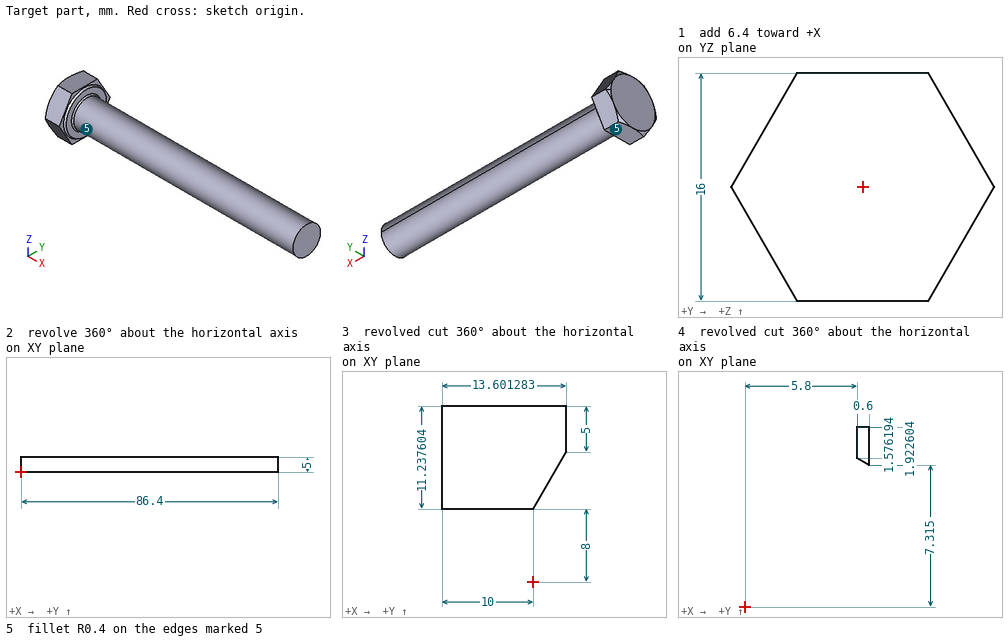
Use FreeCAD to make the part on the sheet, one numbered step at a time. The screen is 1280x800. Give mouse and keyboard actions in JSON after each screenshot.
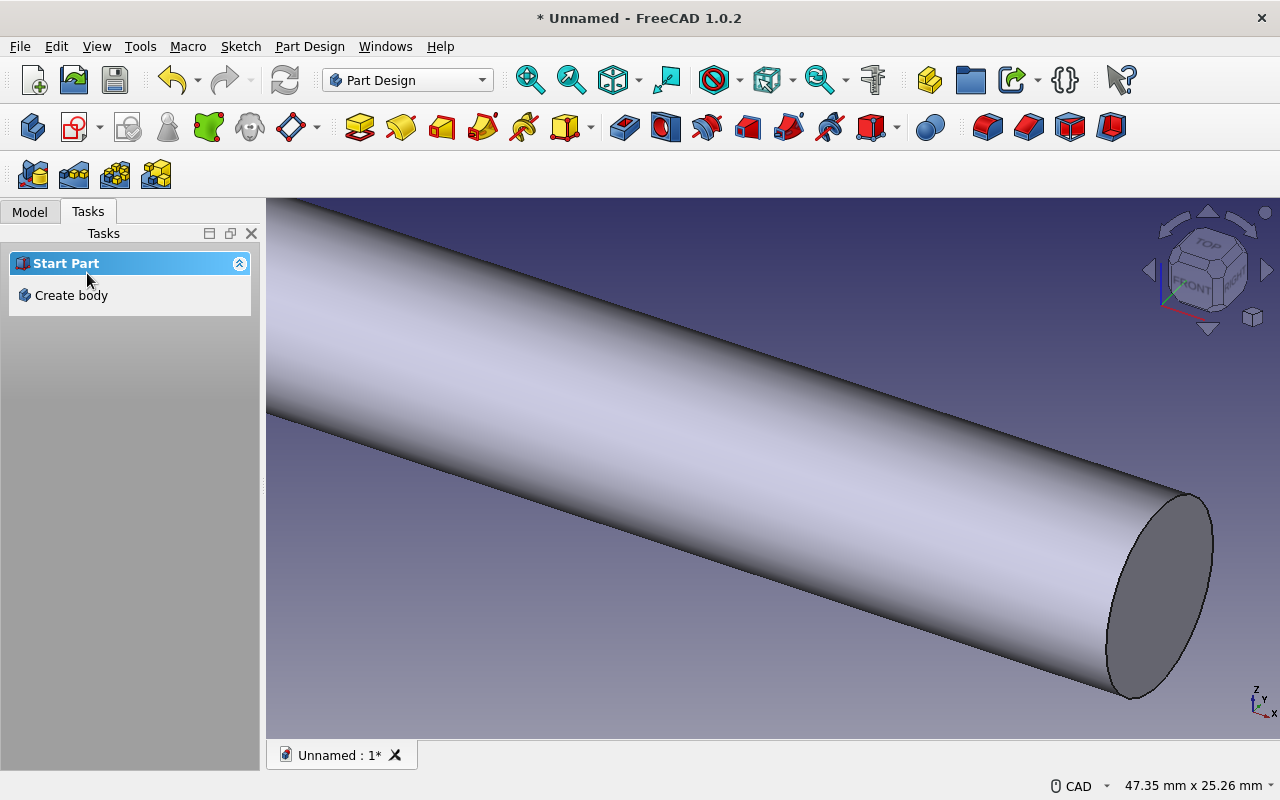
{"action": "key", "text": "v f"}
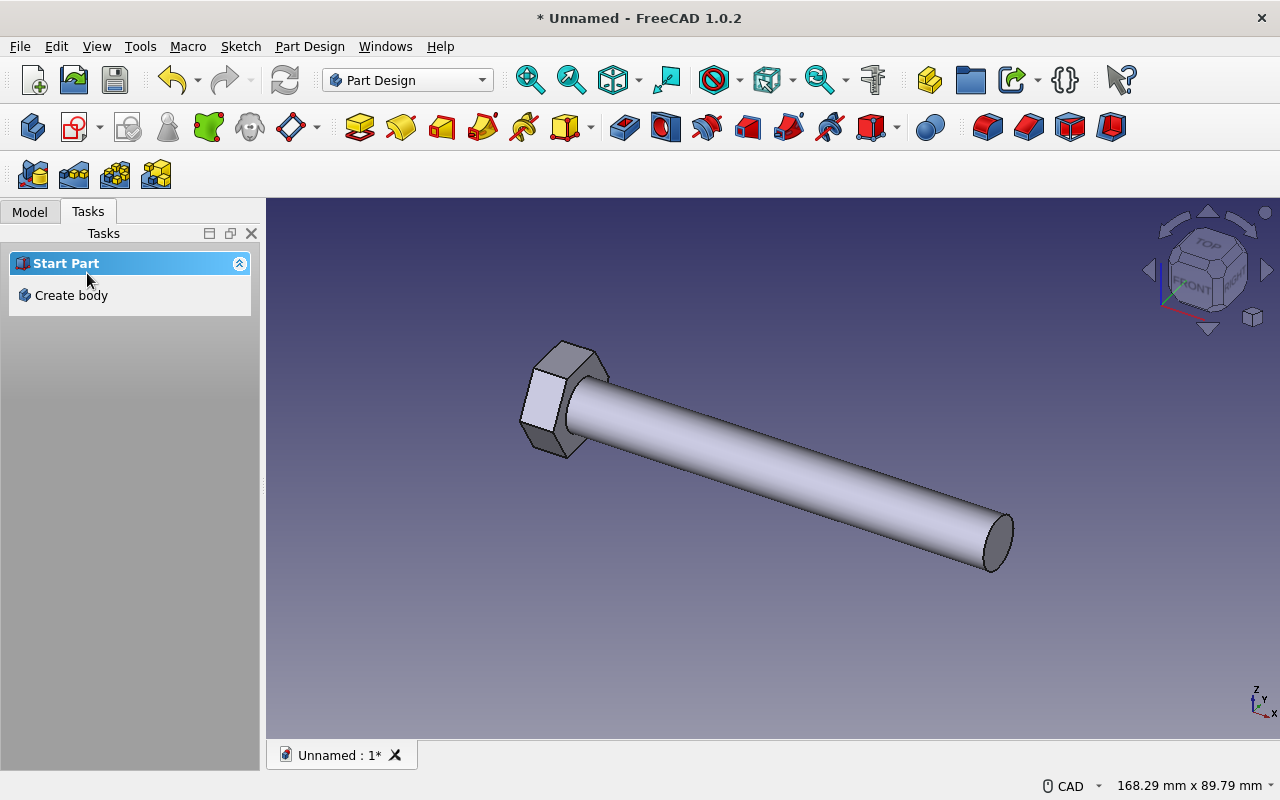
{"action": "left_click", "coordinate": [74, 128]}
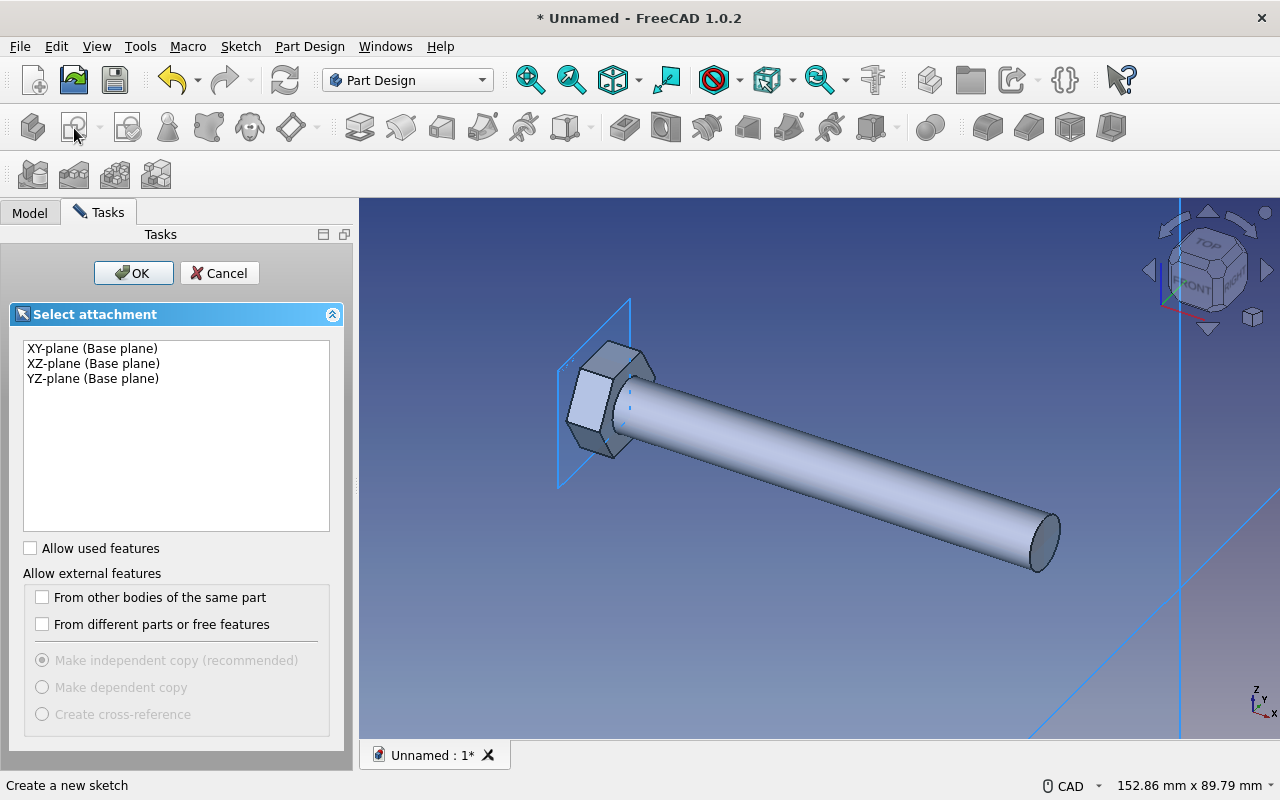
{"action": "left_click", "coordinate": [84, 348]}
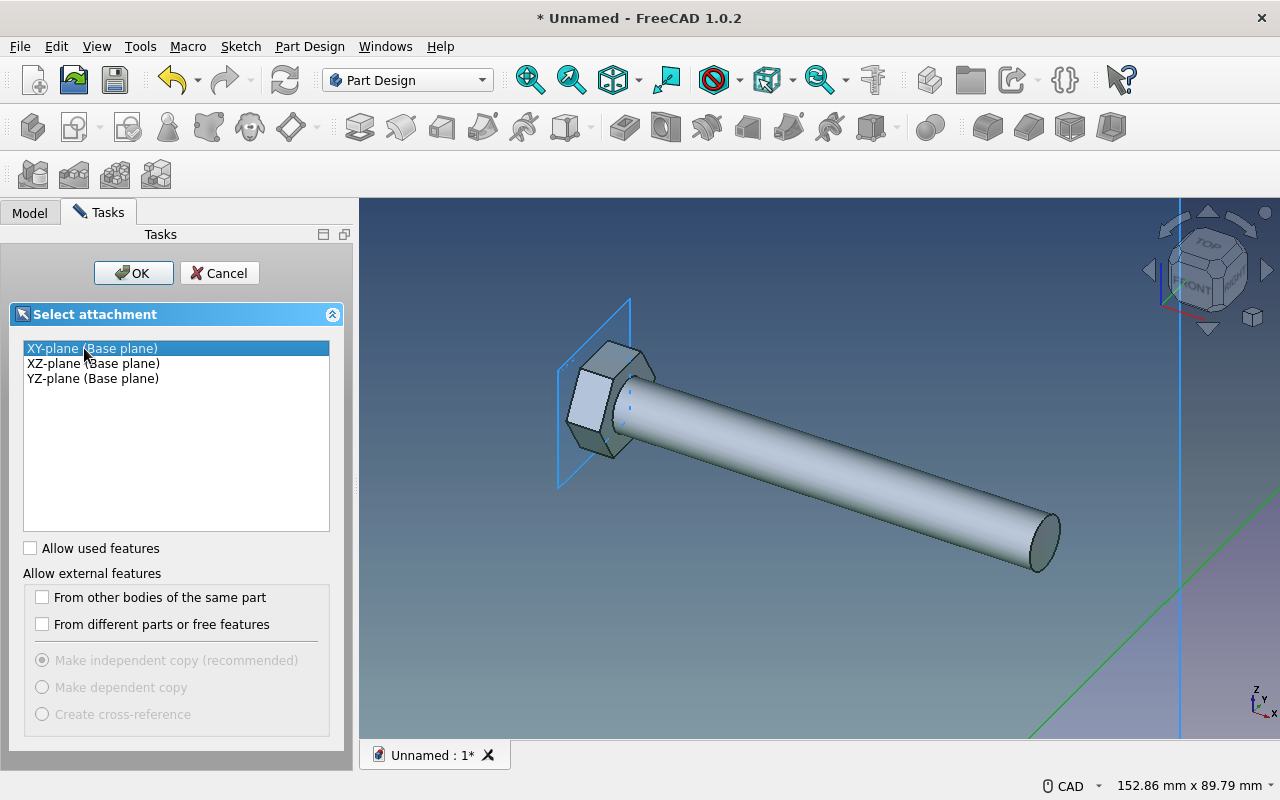
{"action": "left_click", "coordinate": [134, 273]}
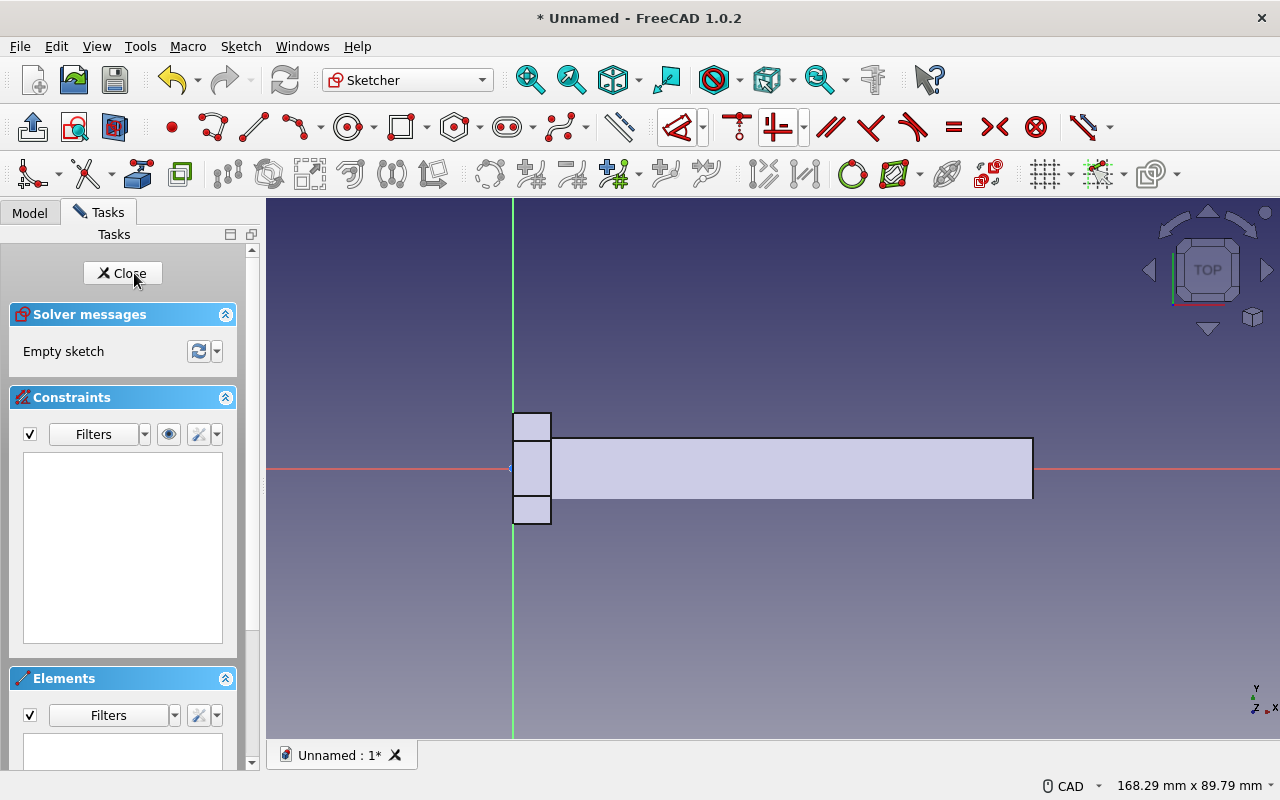
{"action": "left_click", "coordinate": [115, 128]}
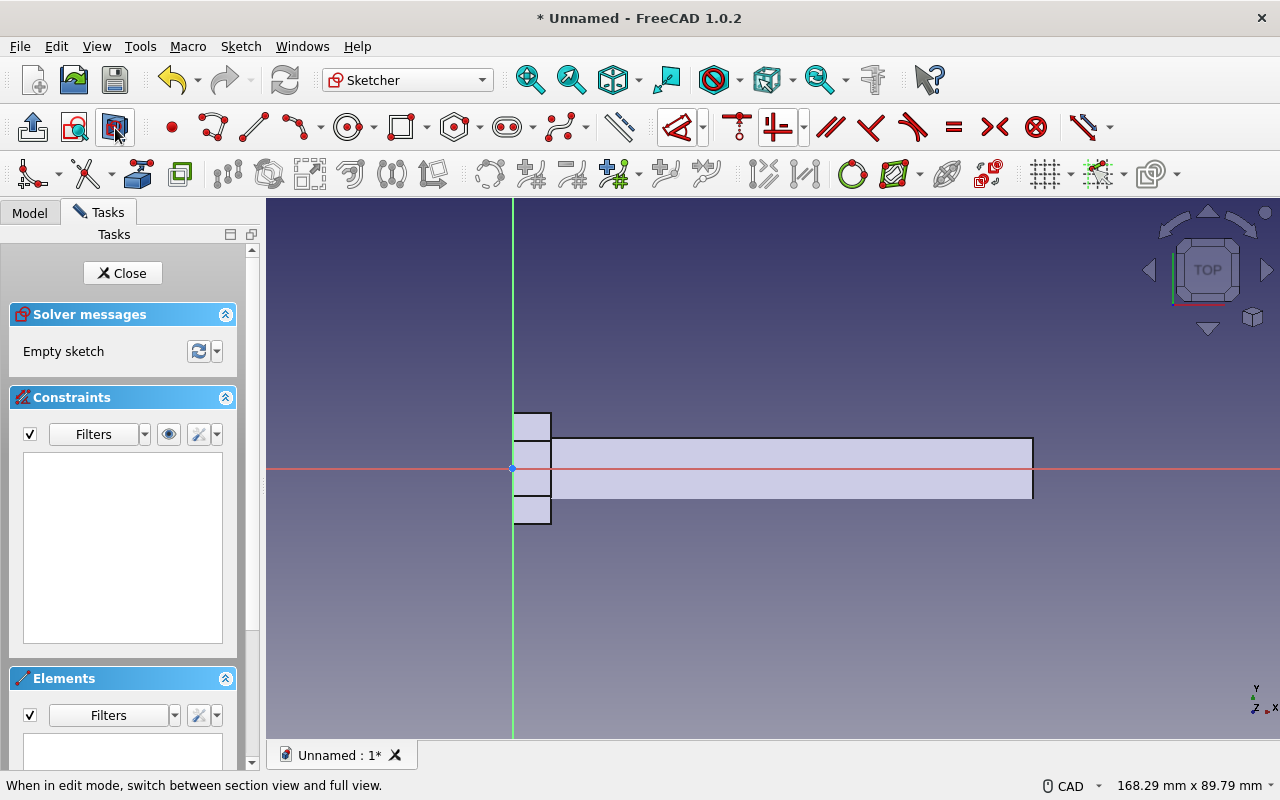
{"action": "scroll", "coordinate": [371, 377], "scroll_direction": "up", "scroll_amount": 5}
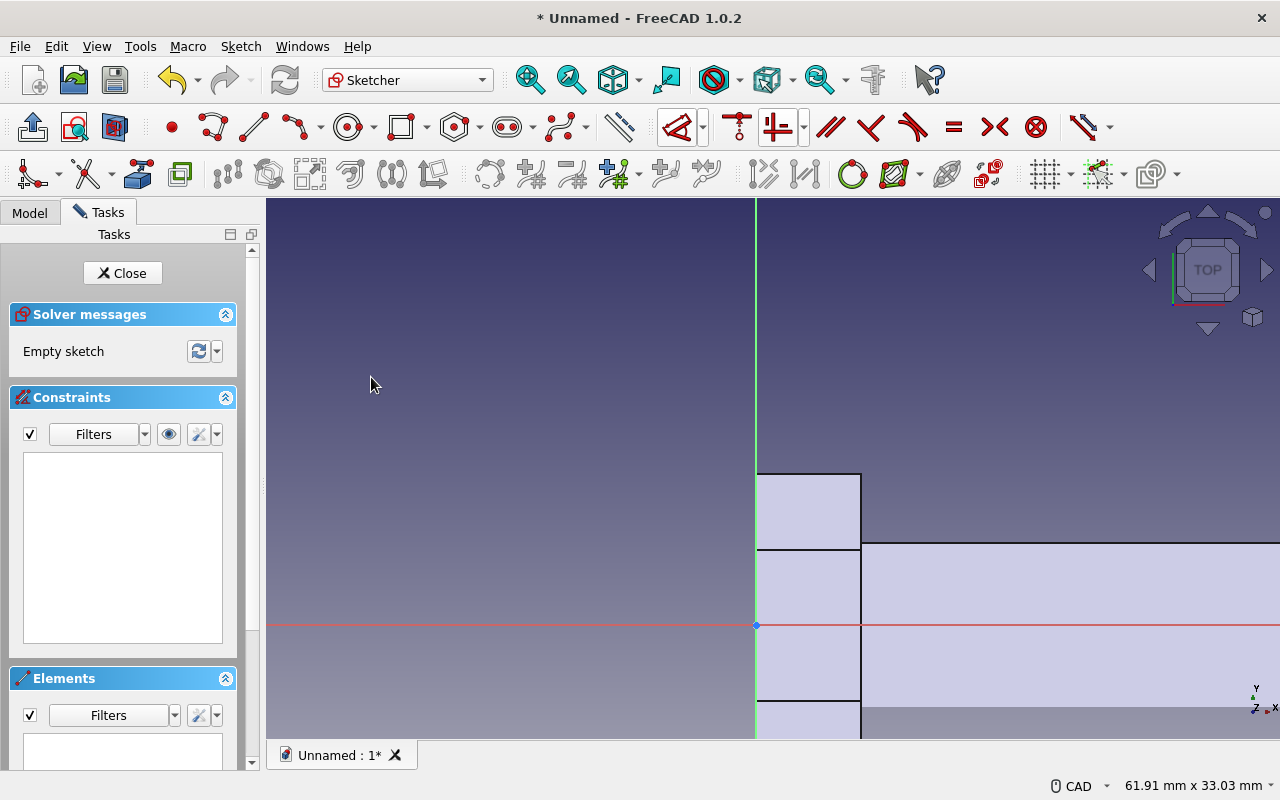
{"action": "left_click", "coordinate": [213, 128]}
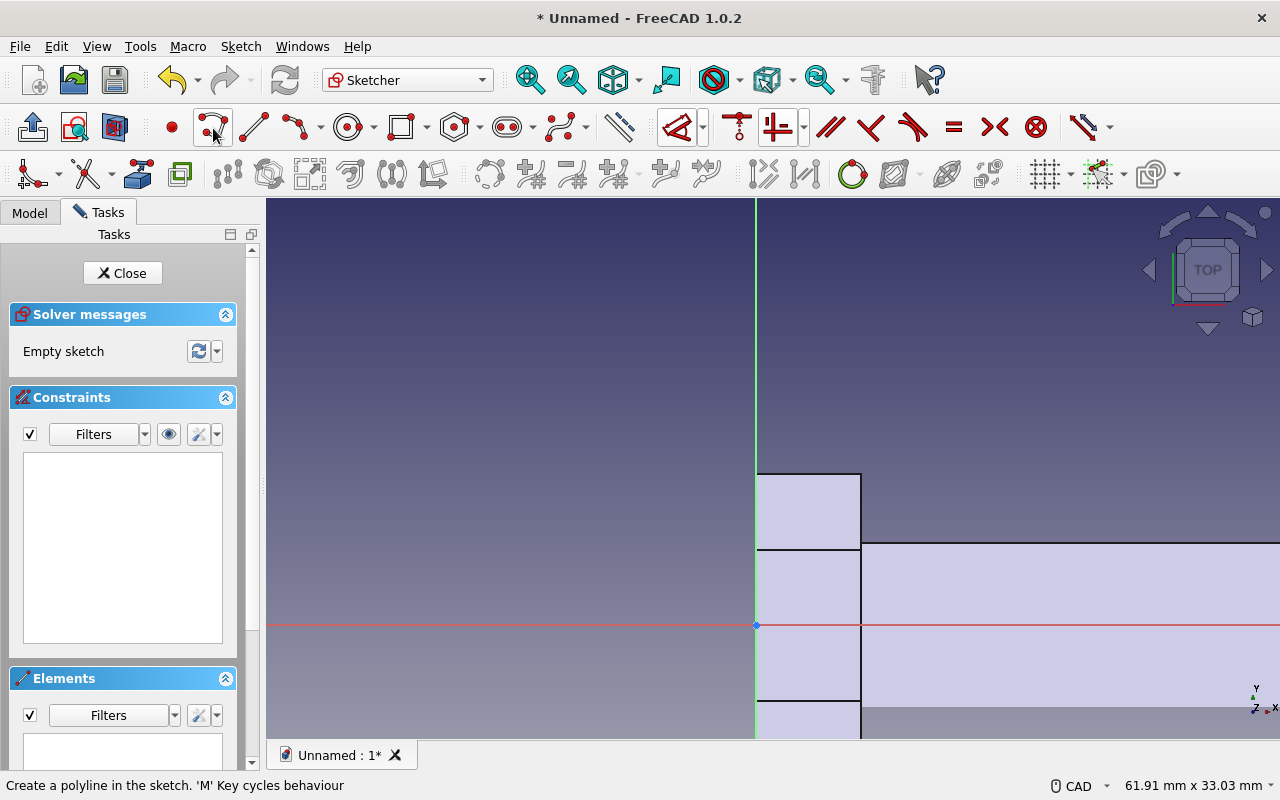
{"action": "left_click", "coordinate": [756, 494]}
{"action": "left_click", "coordinate": [815, 392]}
{"action": "left_click", "coordinate": [815, 310]}
{"action": "left_click", "coordinate": [592, 310]}
{"action": "left_click", "coordinate": [592, 494]}
{"action": "left_click", "coordinate": [756, 495]}
{"action": "key", "text": "Escape"}
{"action": "key", "text": "Escape"}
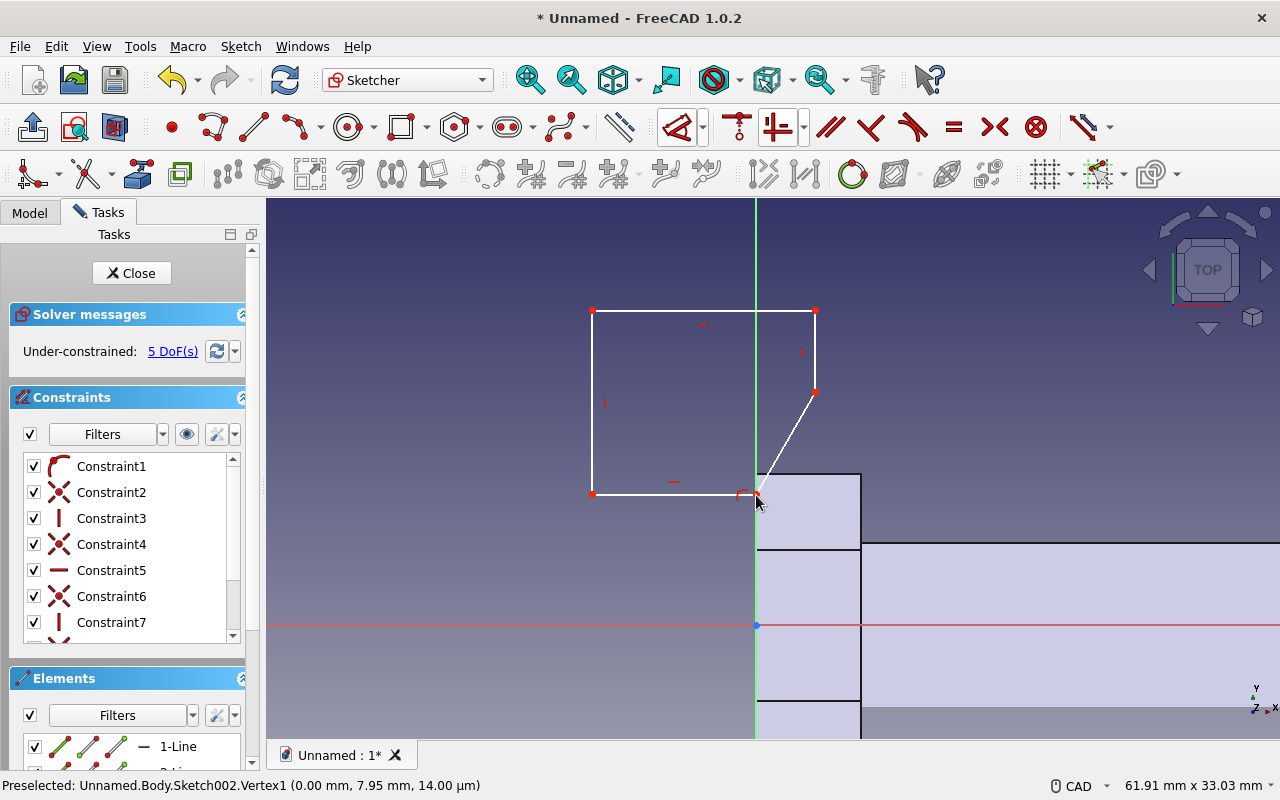
{"action": "left_click", "coordinate": [815, 368]}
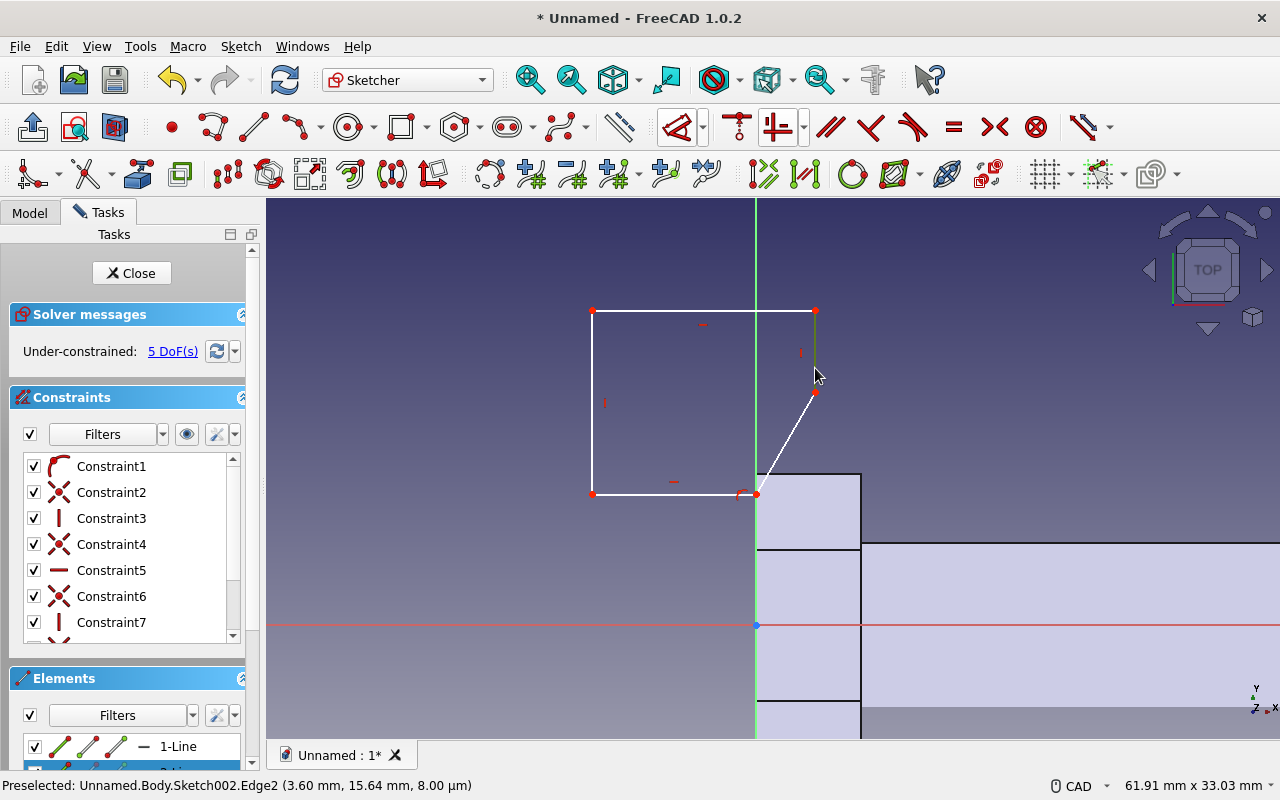
{"action": "key", "text": "i"}